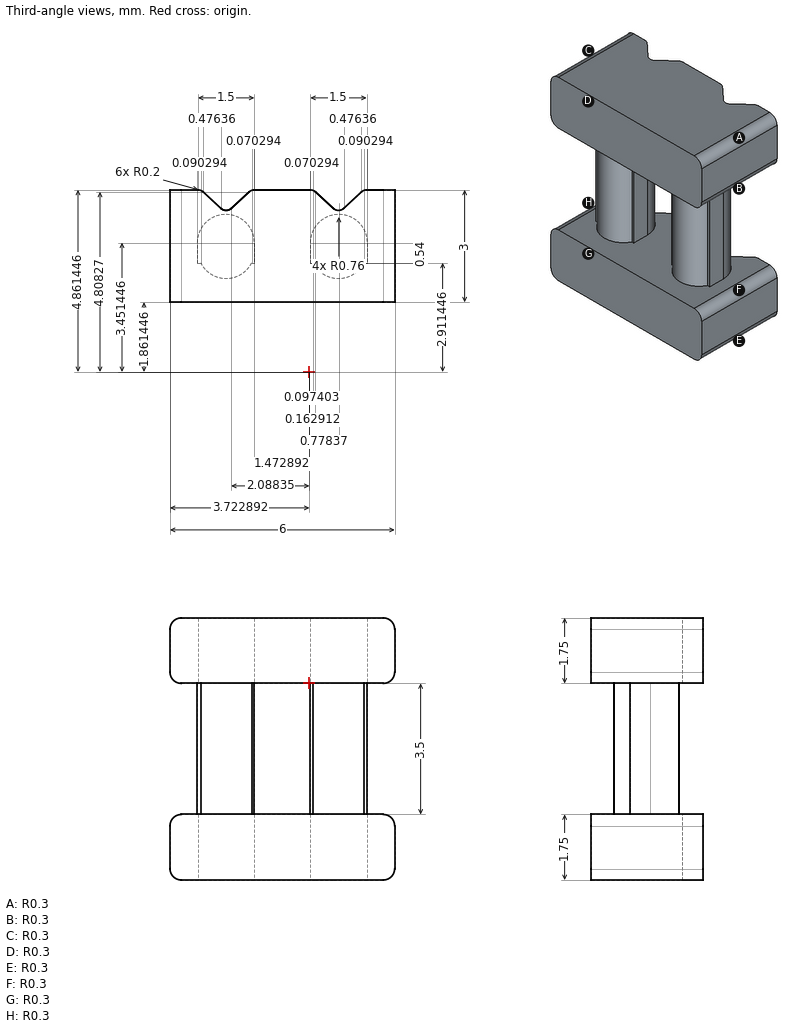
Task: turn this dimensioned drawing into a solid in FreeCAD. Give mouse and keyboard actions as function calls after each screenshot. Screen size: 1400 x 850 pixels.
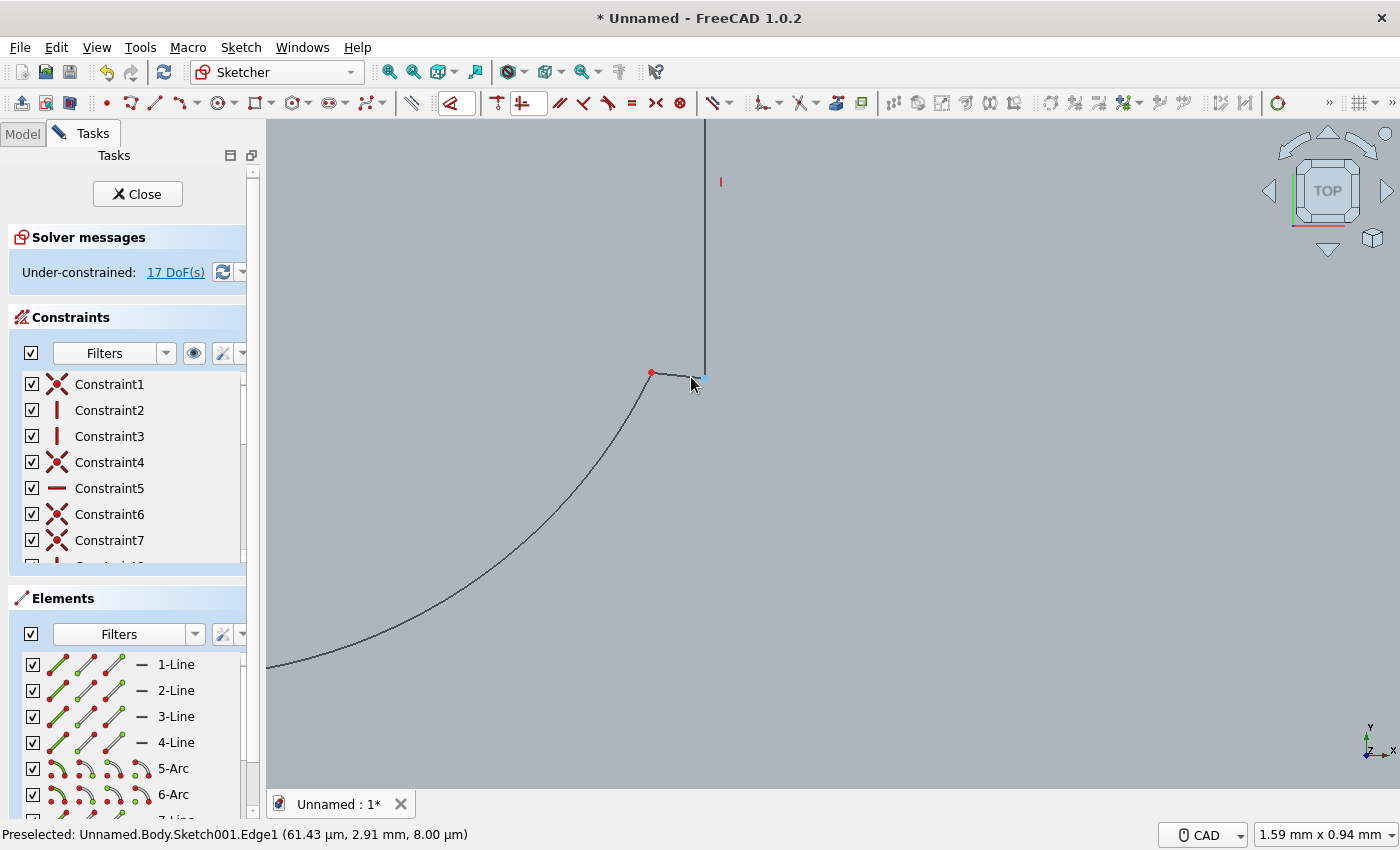
click(689, 377)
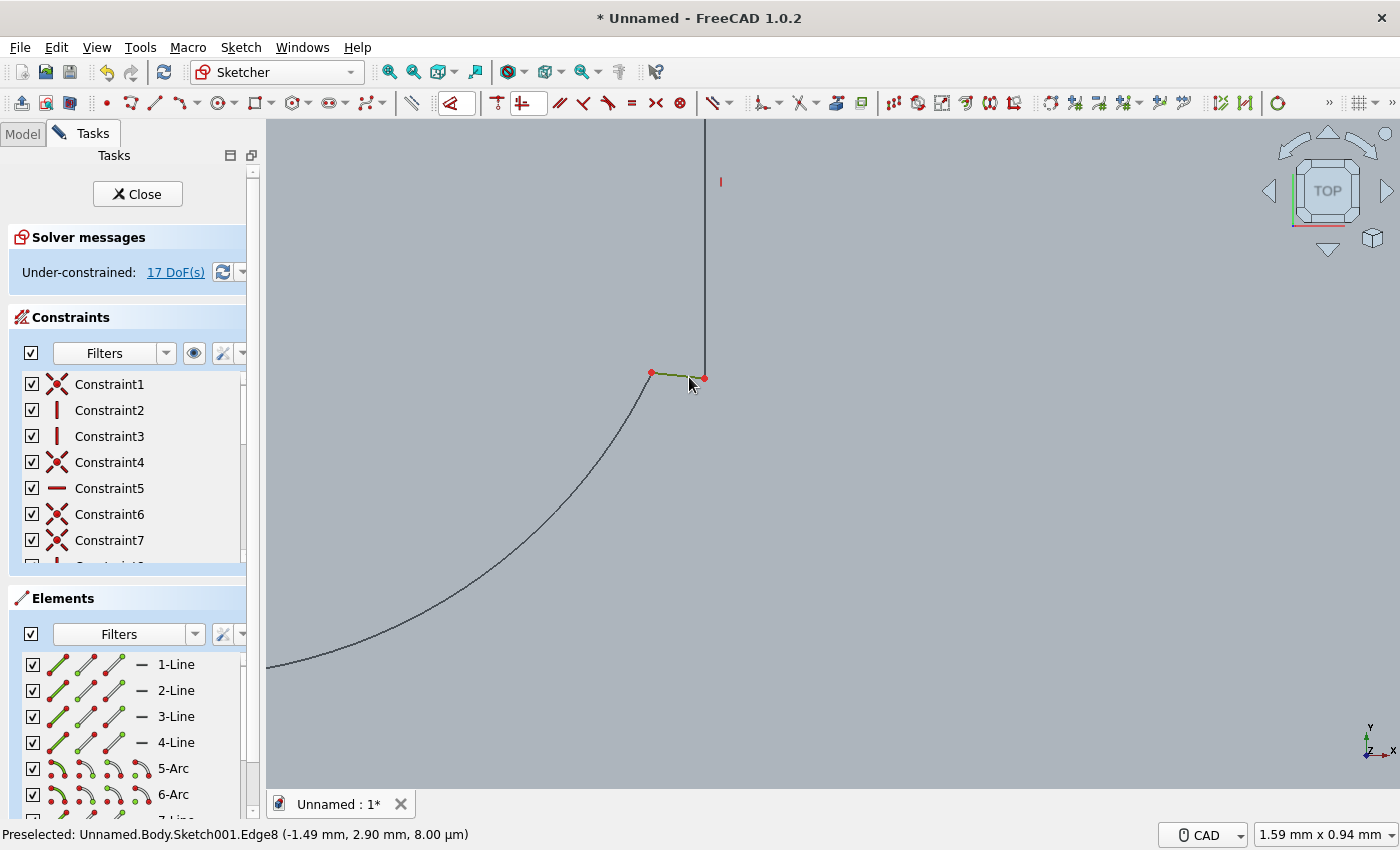
click(542, 104)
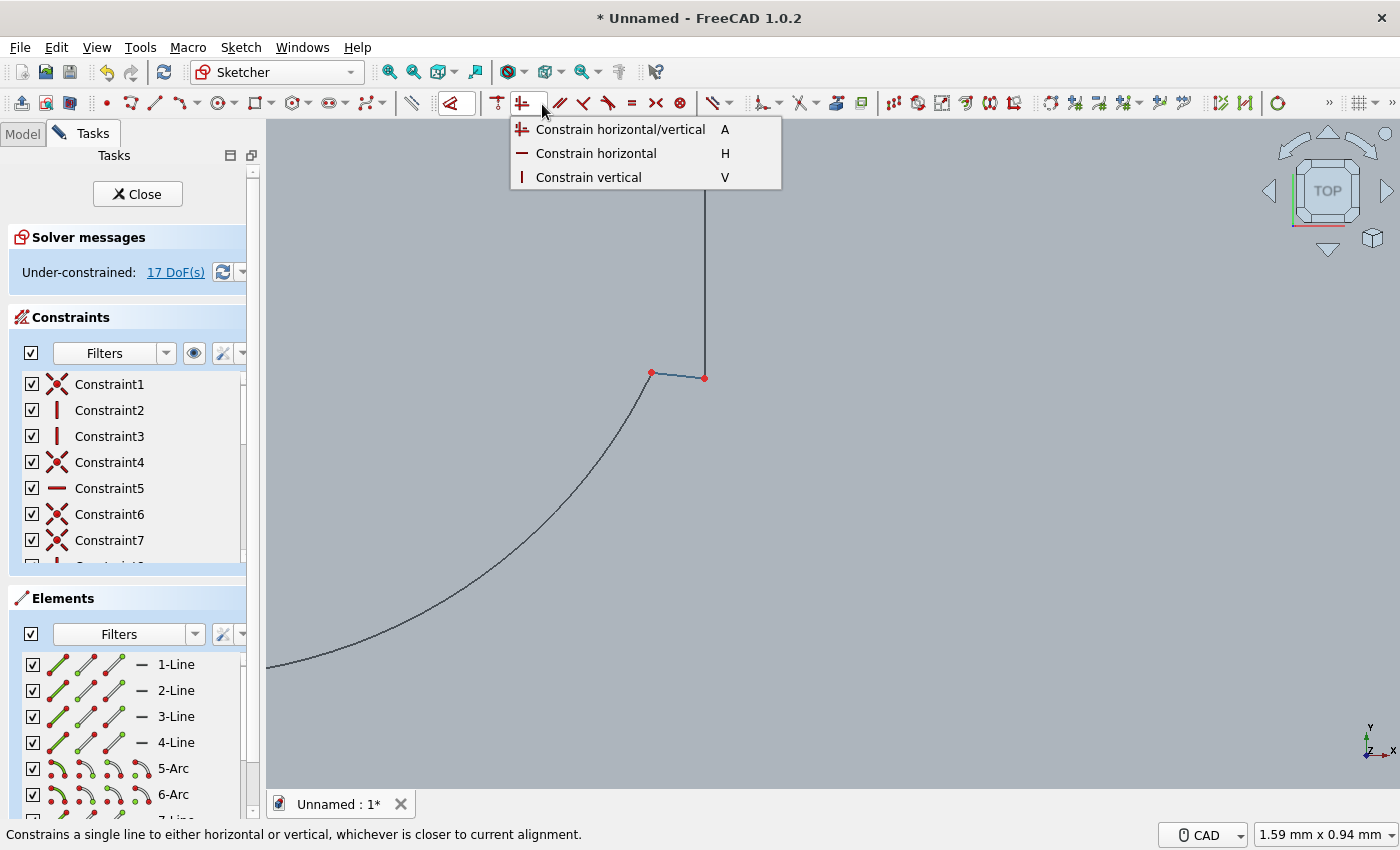
click(646, 153)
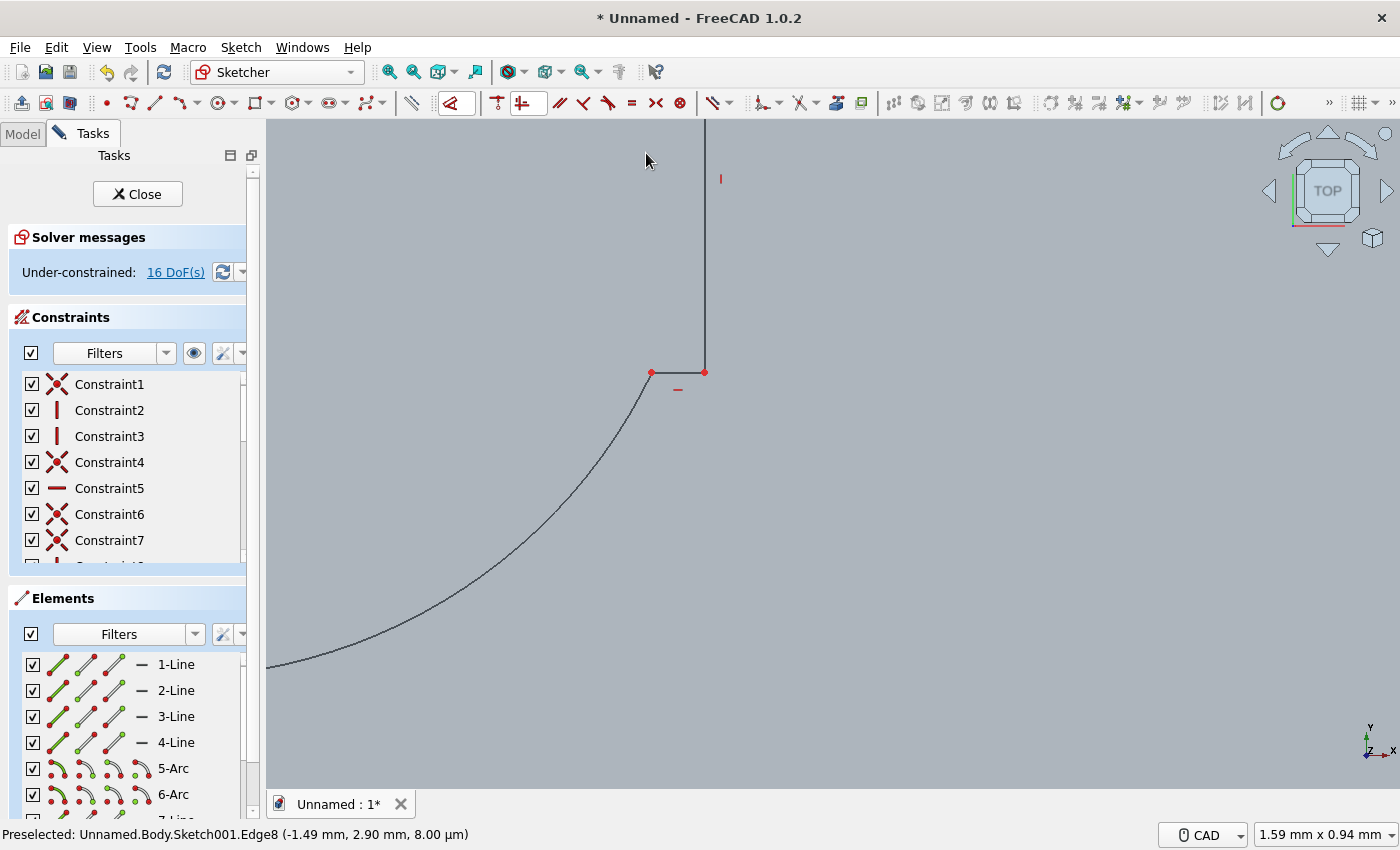
scroll(691, 377, down, 10)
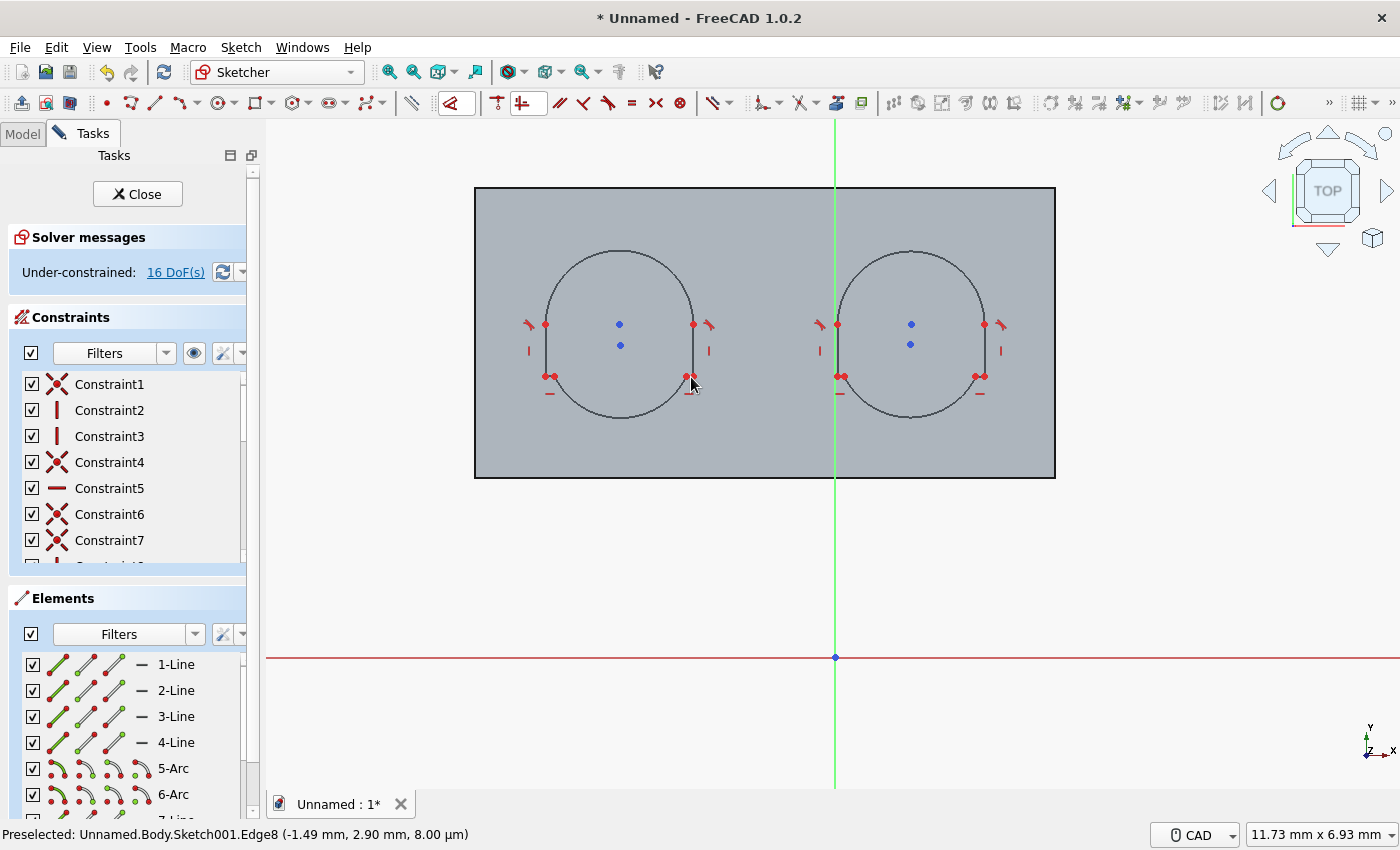
click(954, 265)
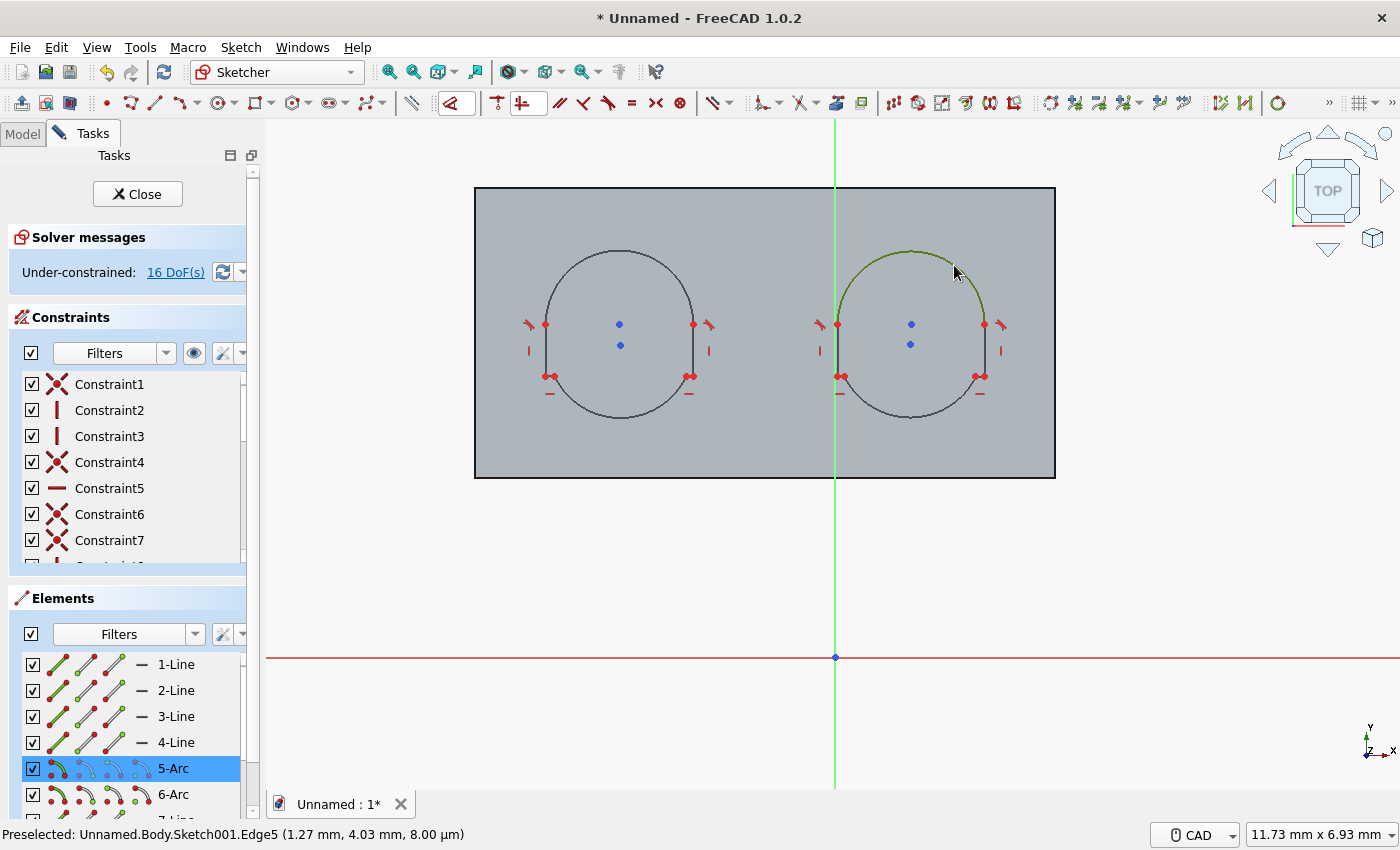
click(878, 410)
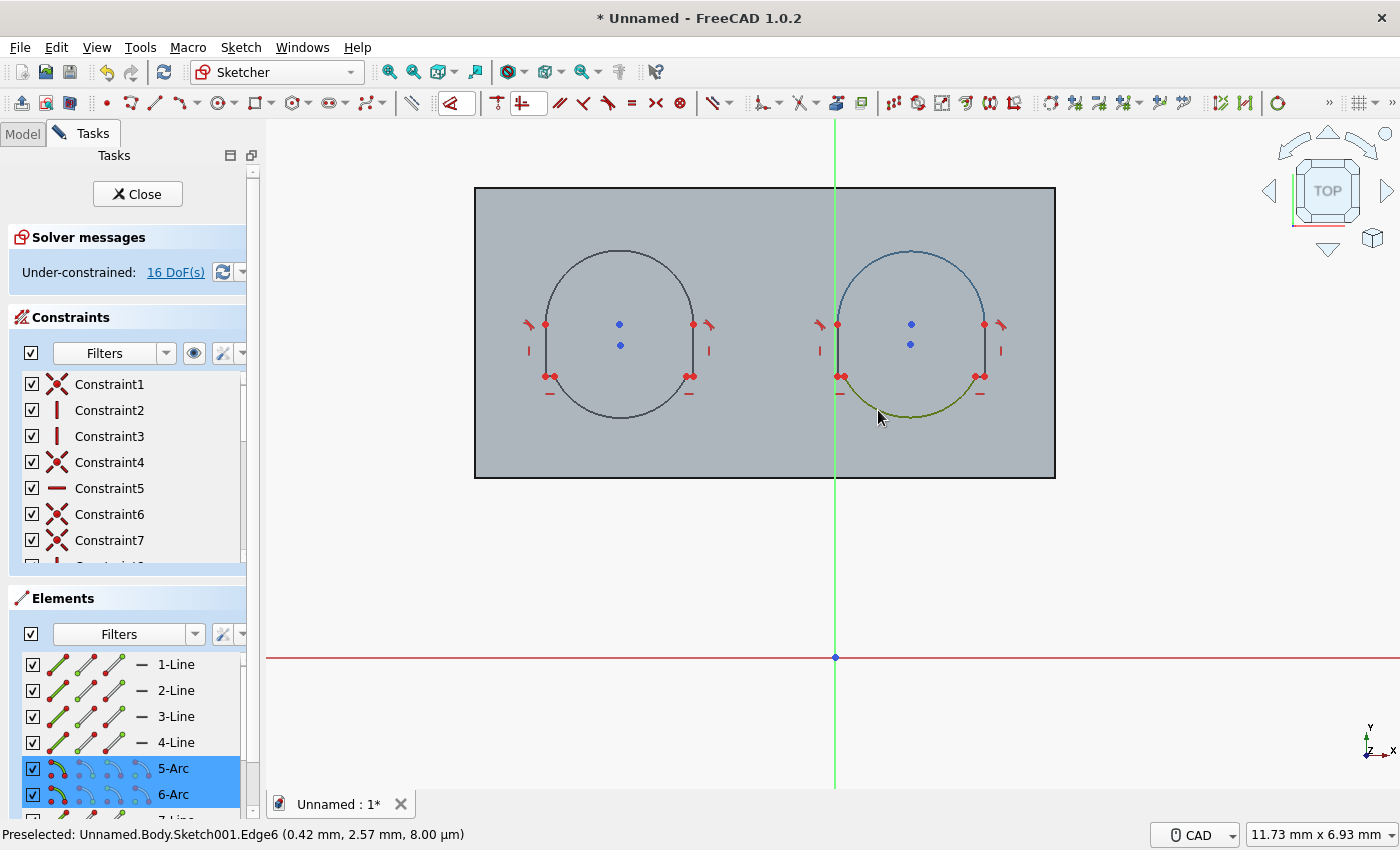
click(589, 411)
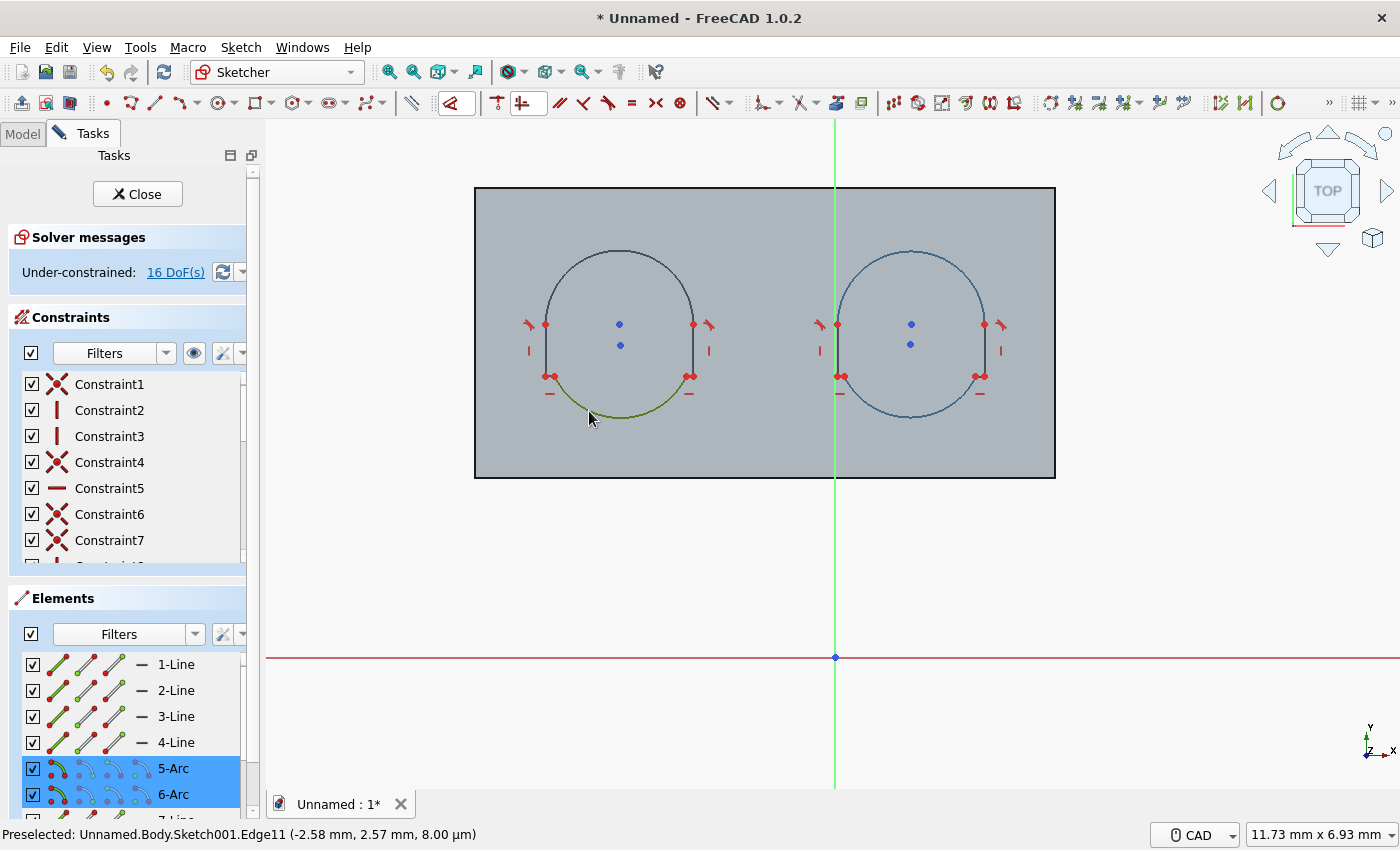
click(663, 265)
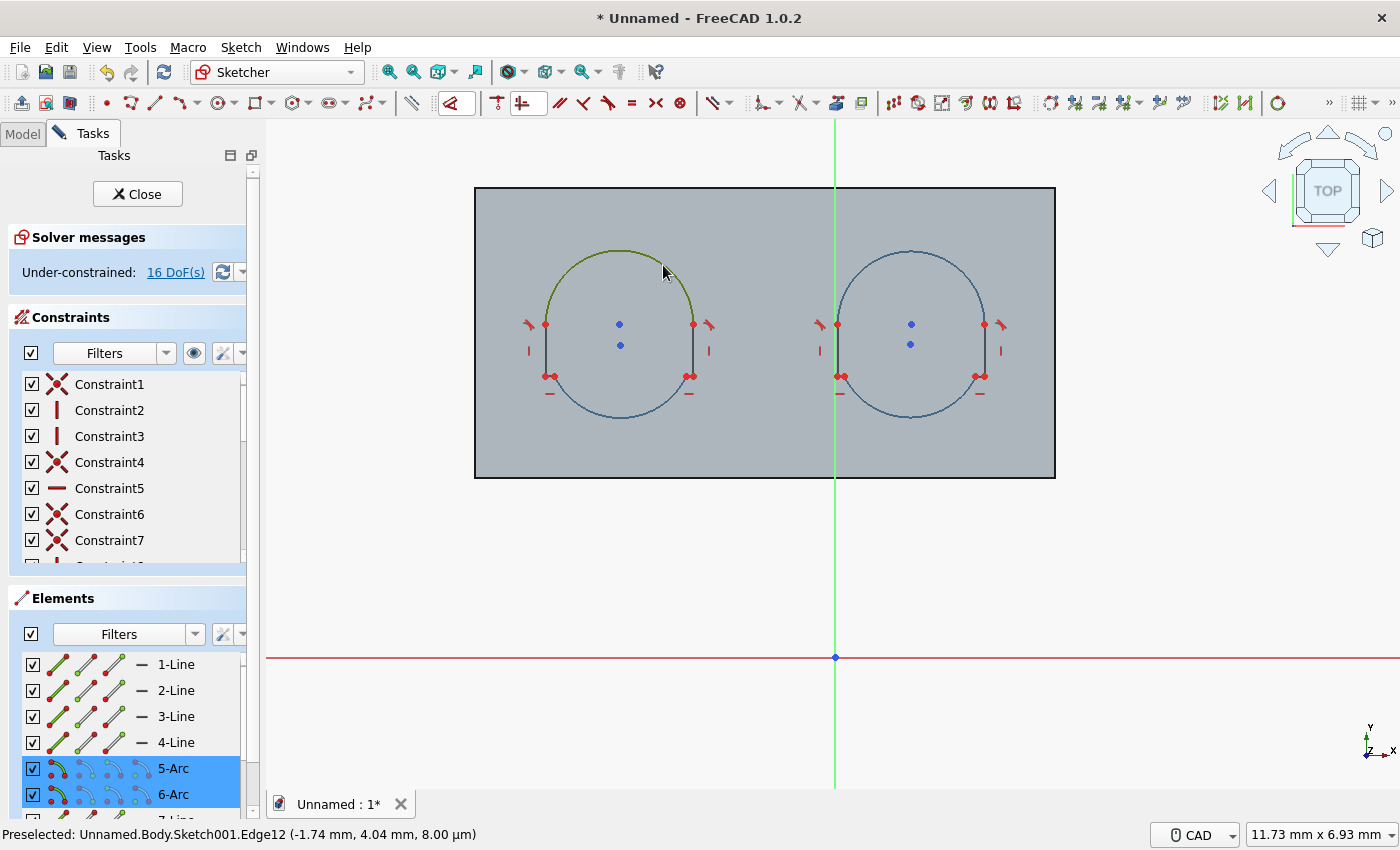
key(e)